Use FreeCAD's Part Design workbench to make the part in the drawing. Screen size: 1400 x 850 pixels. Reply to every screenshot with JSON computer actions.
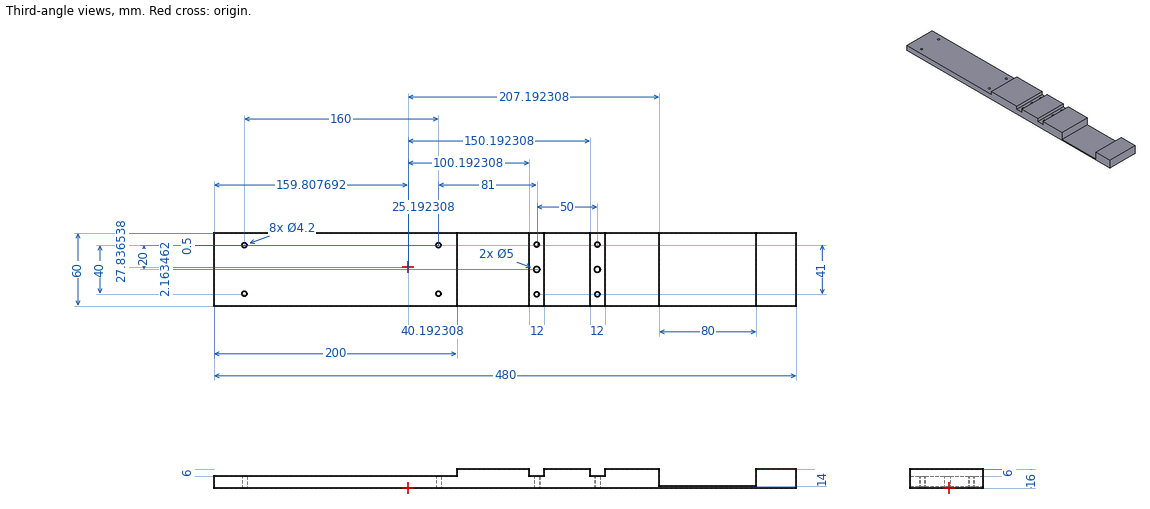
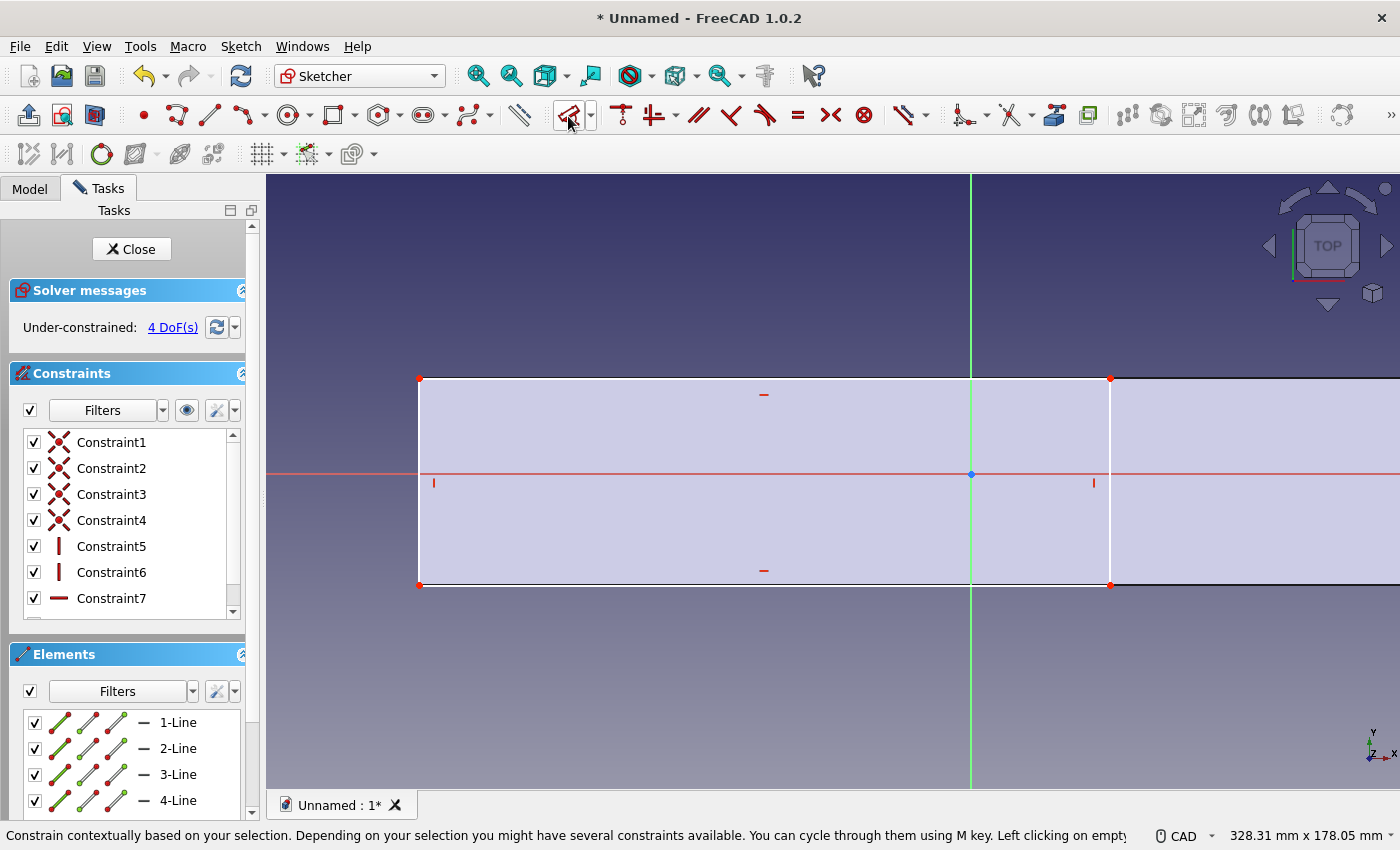
{"action": "left_click", "coordinate": [419, 441]}
{"action": "left_click", "coordinate": [385, 435]}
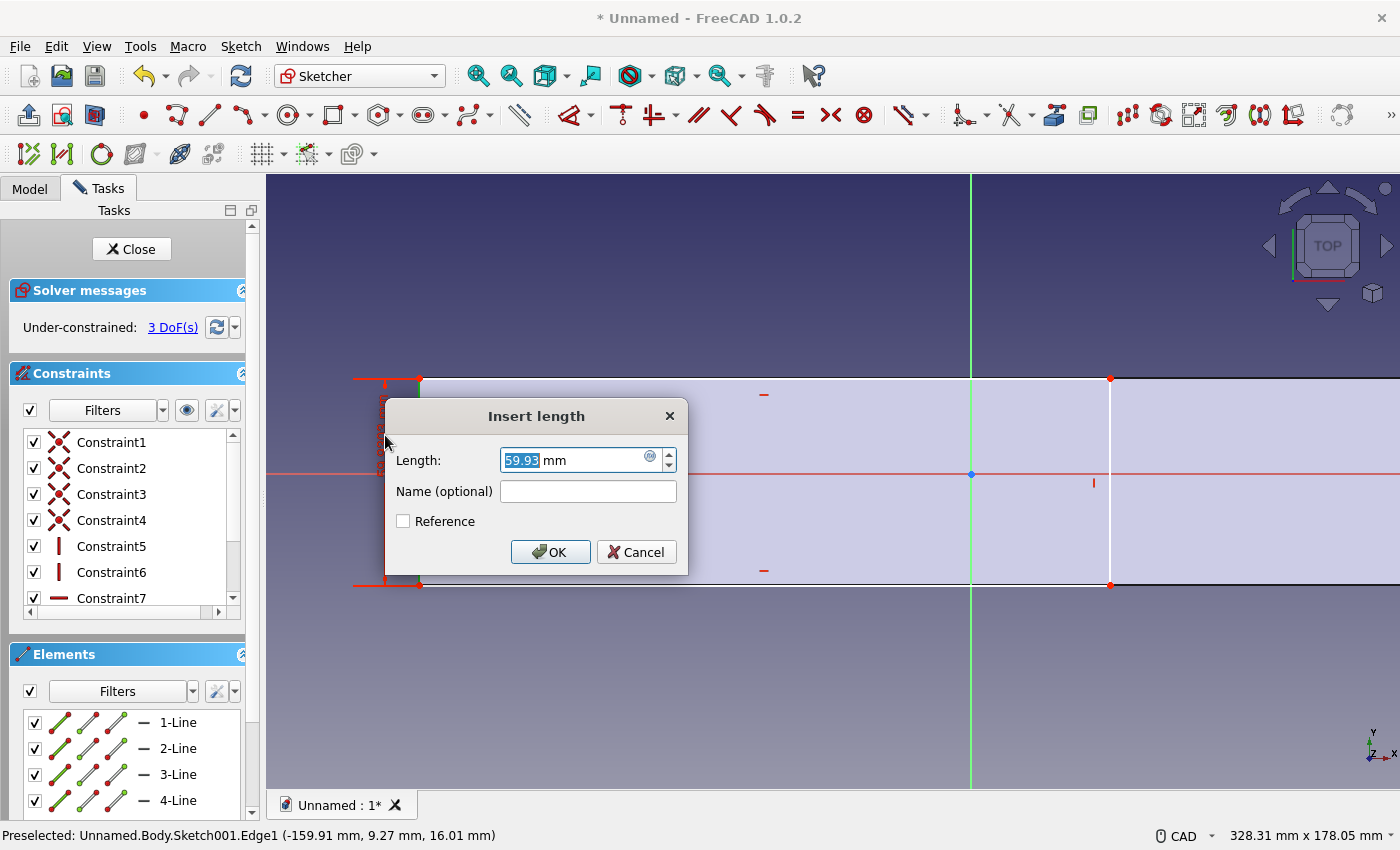
{"action": "type", "text": "60"}
{"action": "key", "text": "Return"}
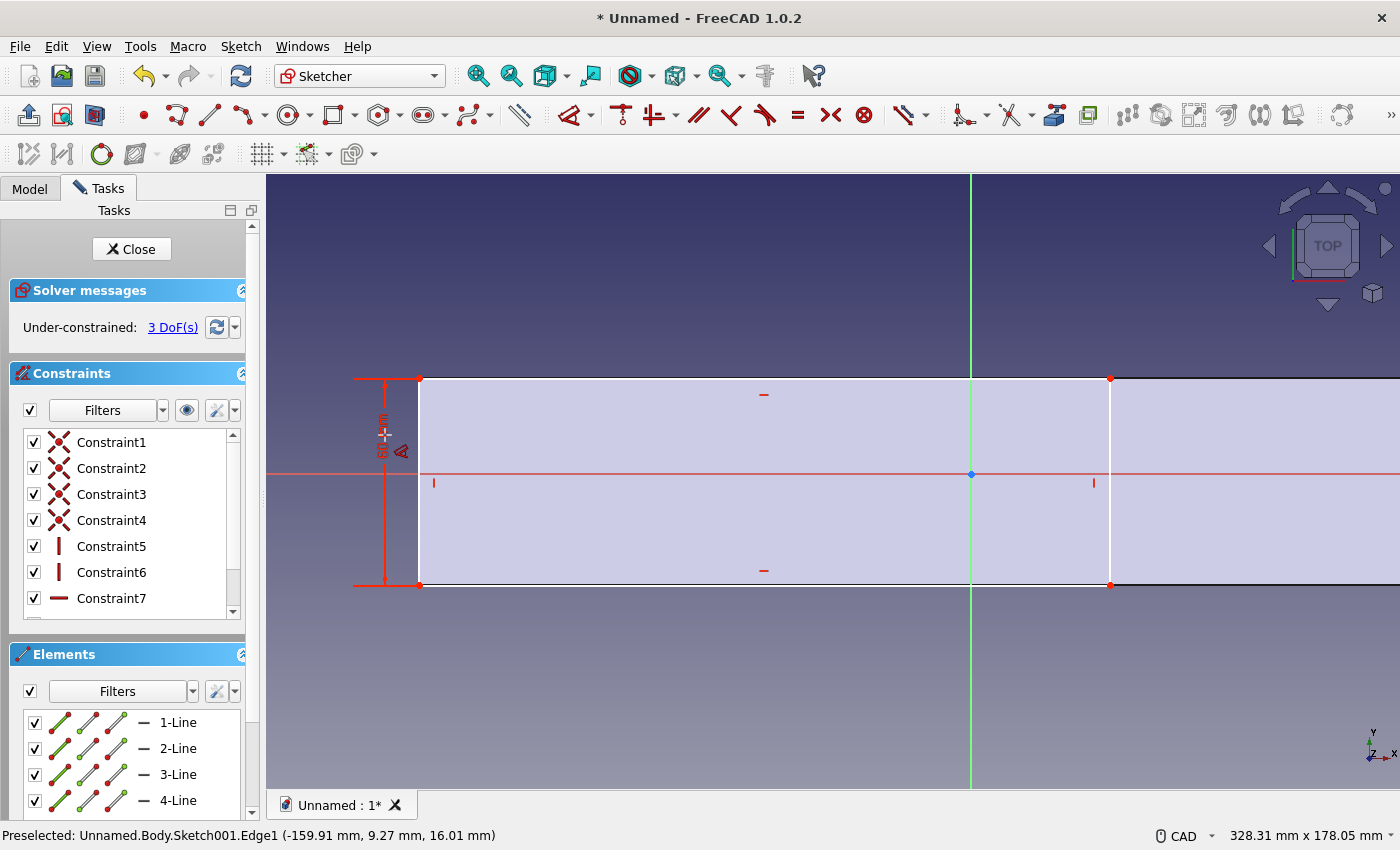
{"action": "left_click", "coordinate": [626, 586]}
{"action": "left_click", "coordinate": [765, 620]}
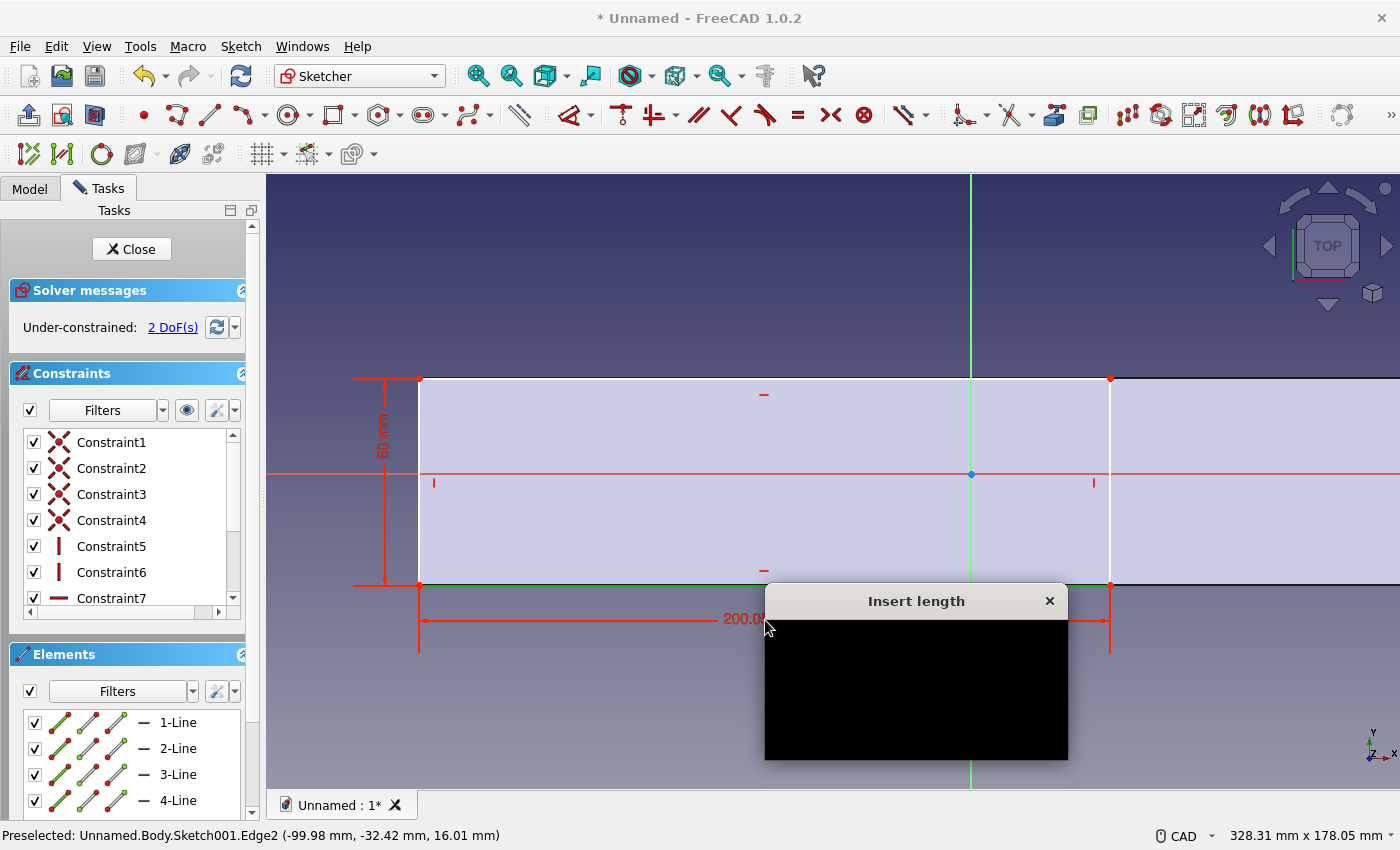
{"action": "type", "text": "200"}
{"action": "key", "text": "Return"}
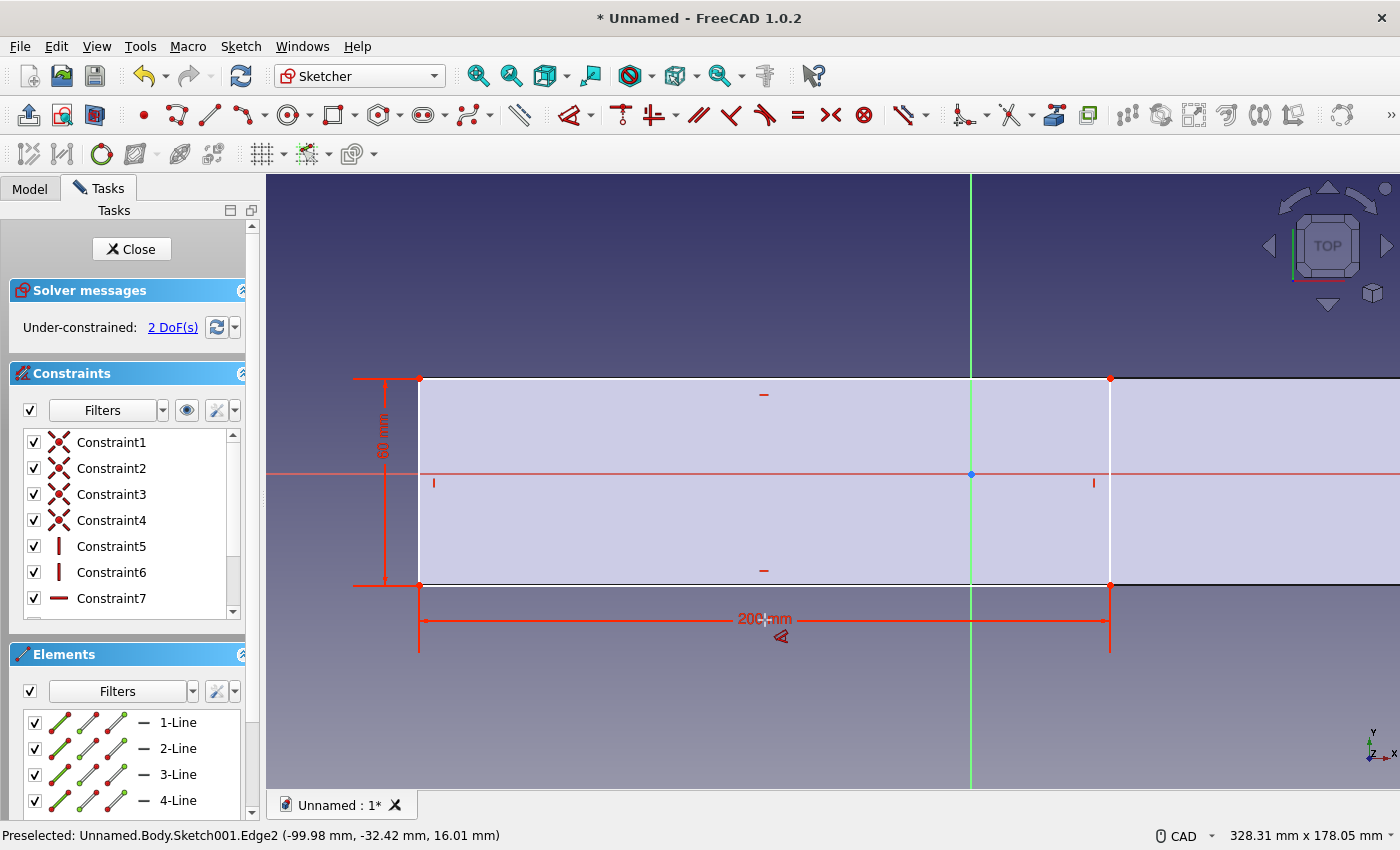
{"action": "left_click", "coordinate": [419, 379]}
{"action": "left_click", "coordinate": [385, 404]}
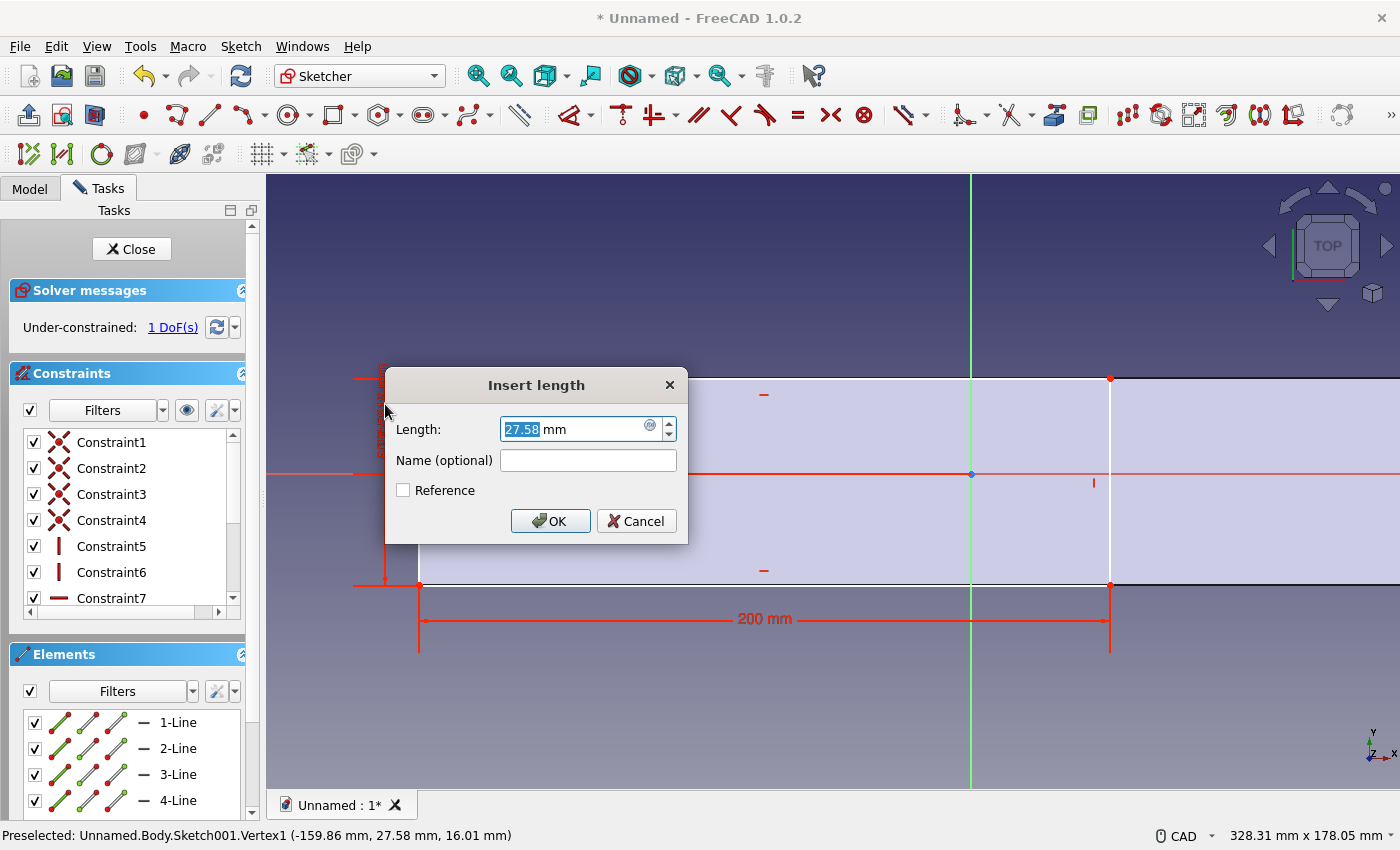
{"action": "type", "text": "27.836538"}
{"action": "key", "text": "Return"}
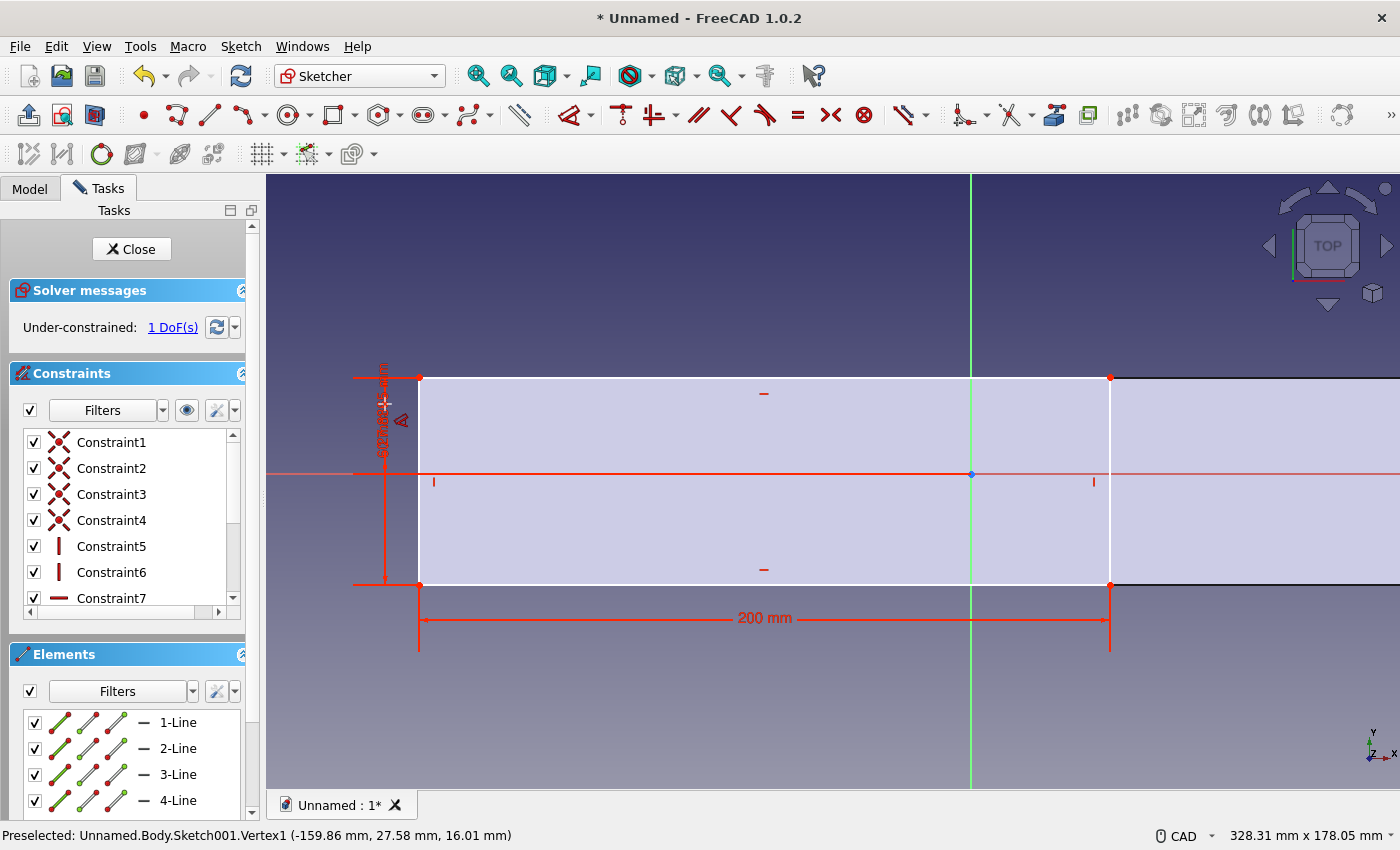
{"action": "left_click", "coordinate": [1110, 585]}
{"action": "left_click", "coordinate": [1041, 619]}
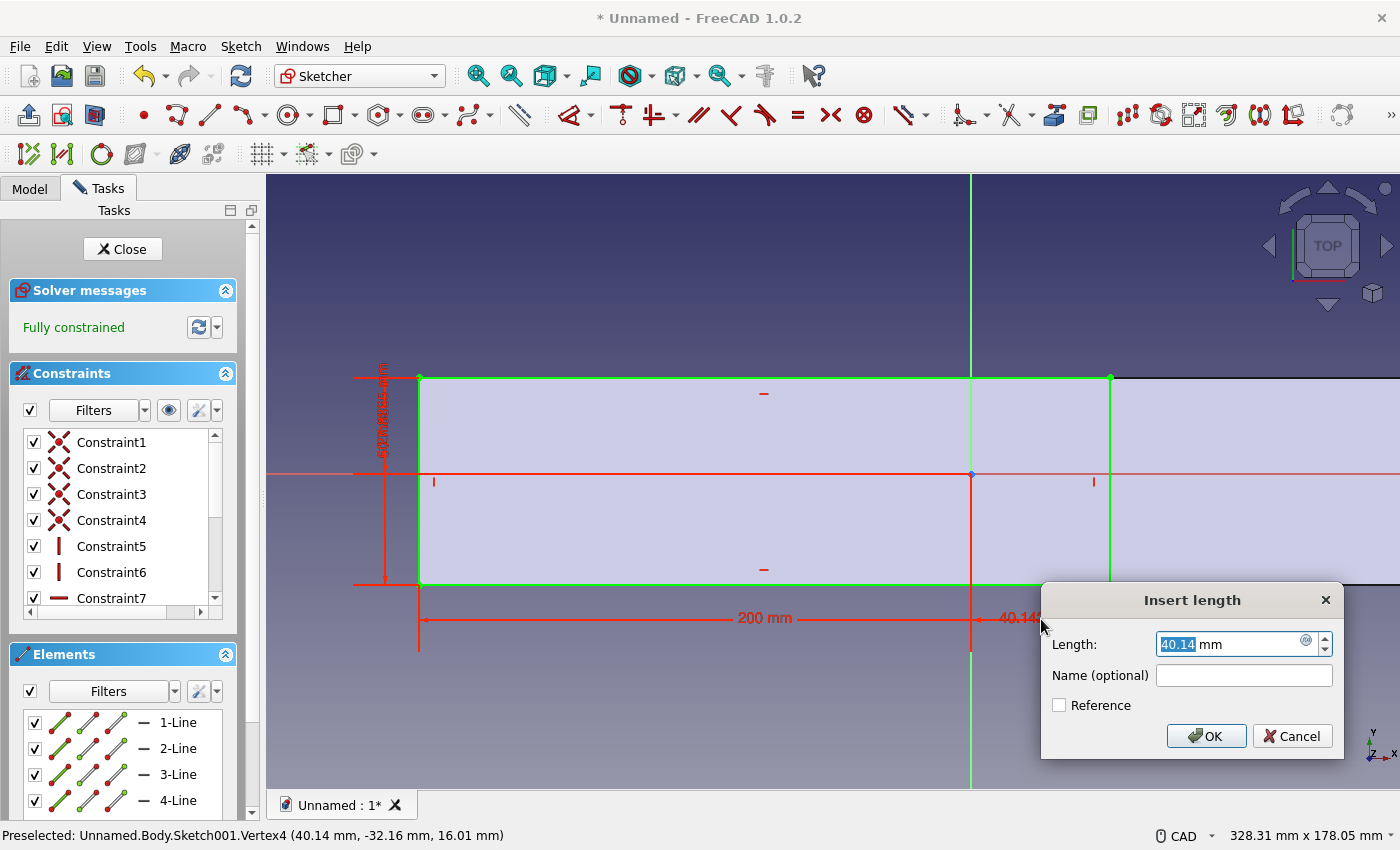
{"action": "type", "text": "40.192308"}
{"action": "key", "text": "Return"}
{"action": "key", "text": "Escape"}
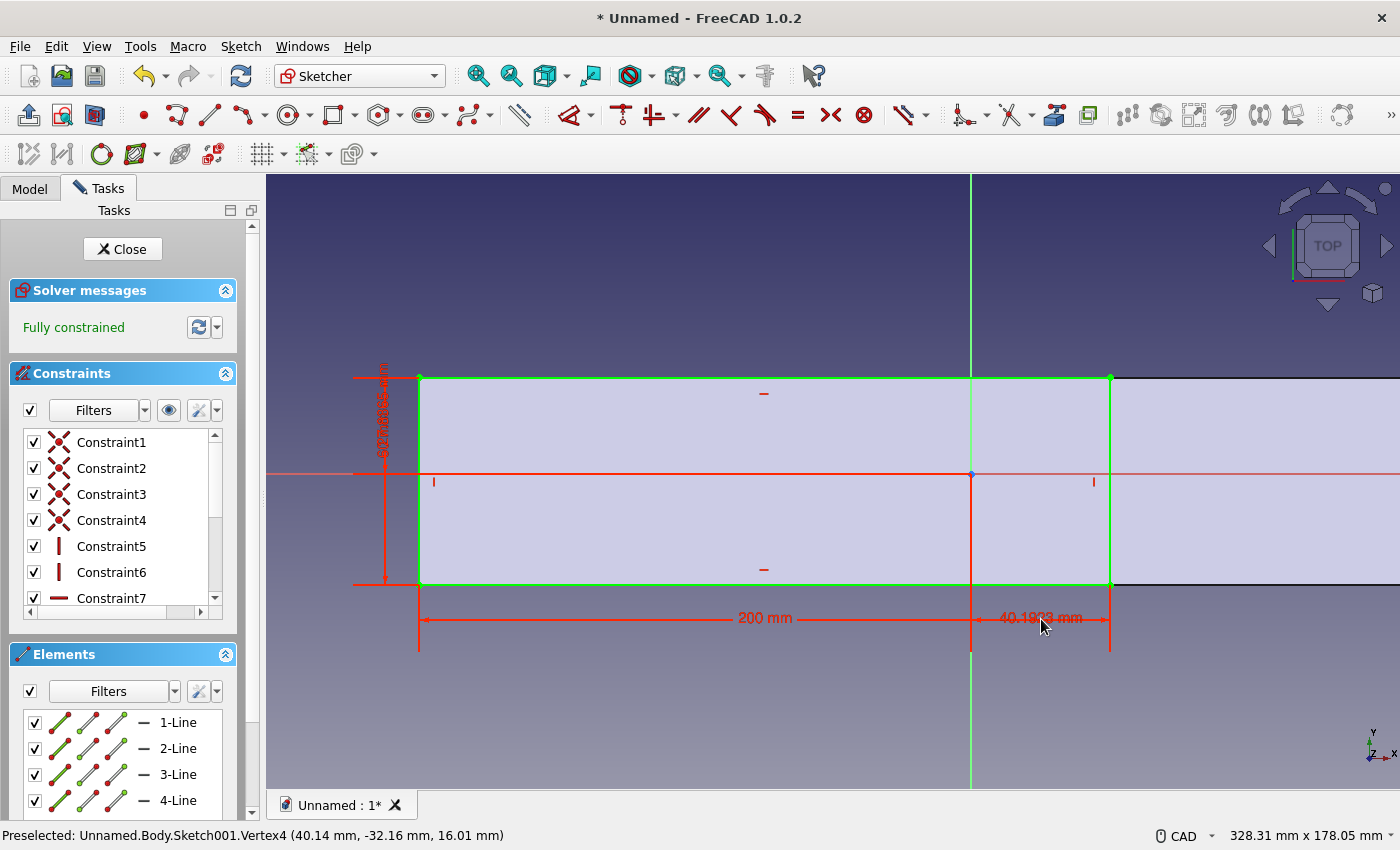
{"action": "left_click", "coordinate": [123, 249]}